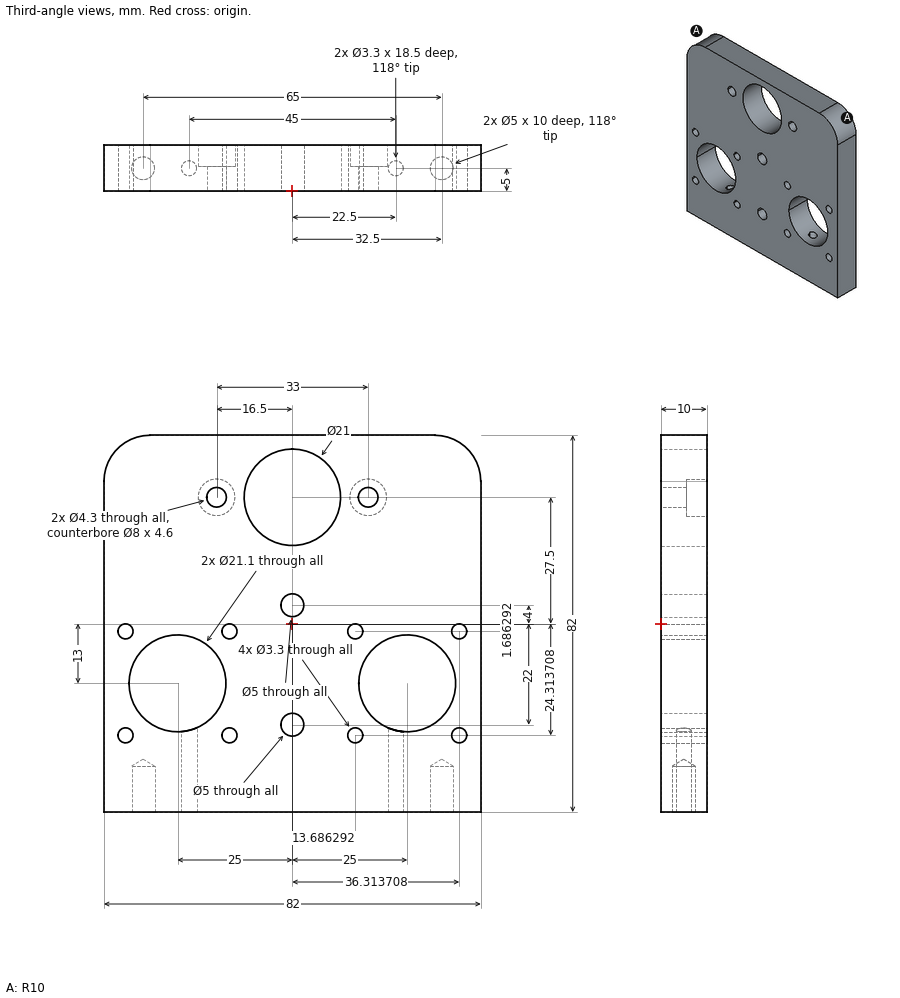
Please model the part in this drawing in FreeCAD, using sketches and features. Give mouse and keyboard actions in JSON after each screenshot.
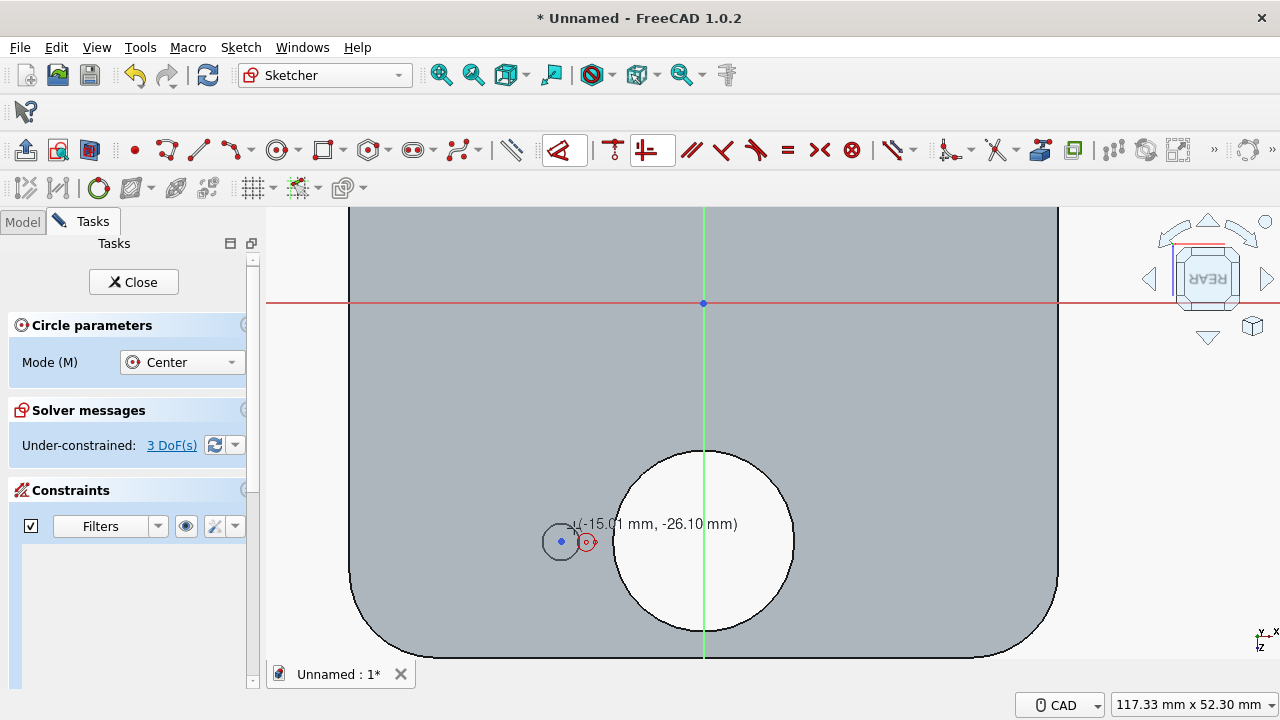
{"action": "left_click", "coordinate": [846, 541]}
{"action": "left_click", "coordinate": [859, 528]}
{"action": "key", "text": "Escape"}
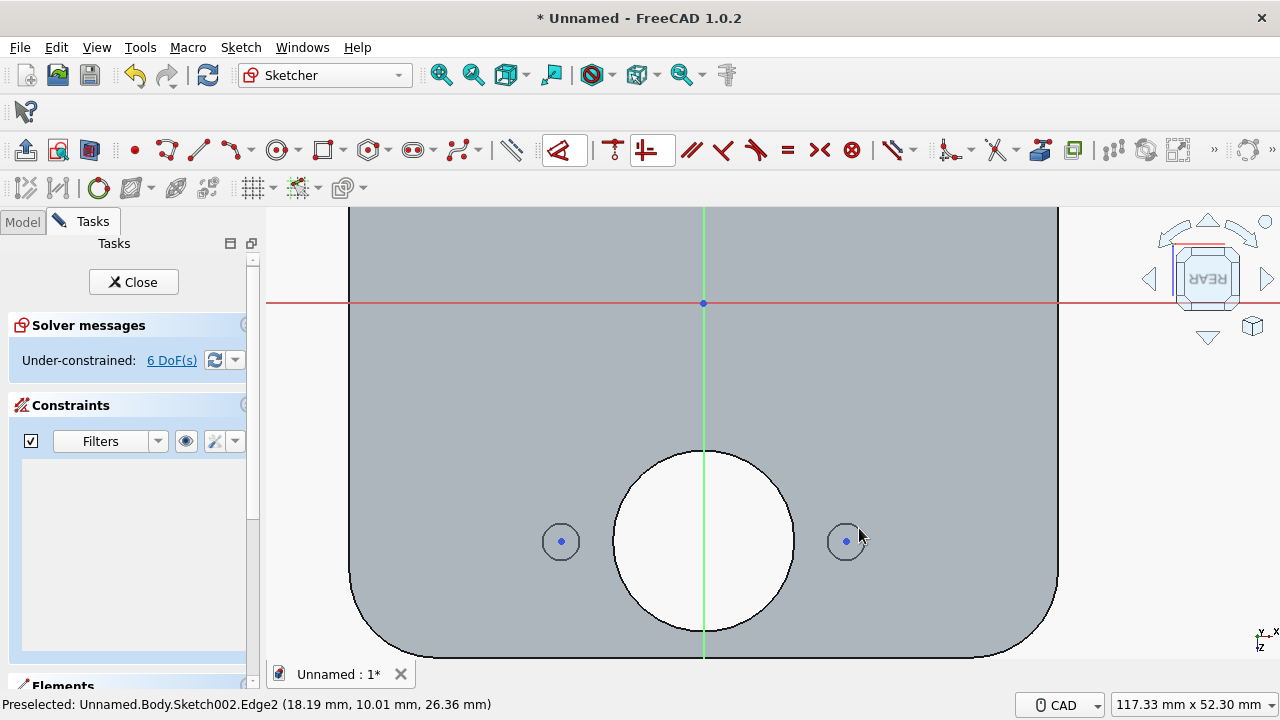
{"action": "left_click", "coordinate": [574, 529]}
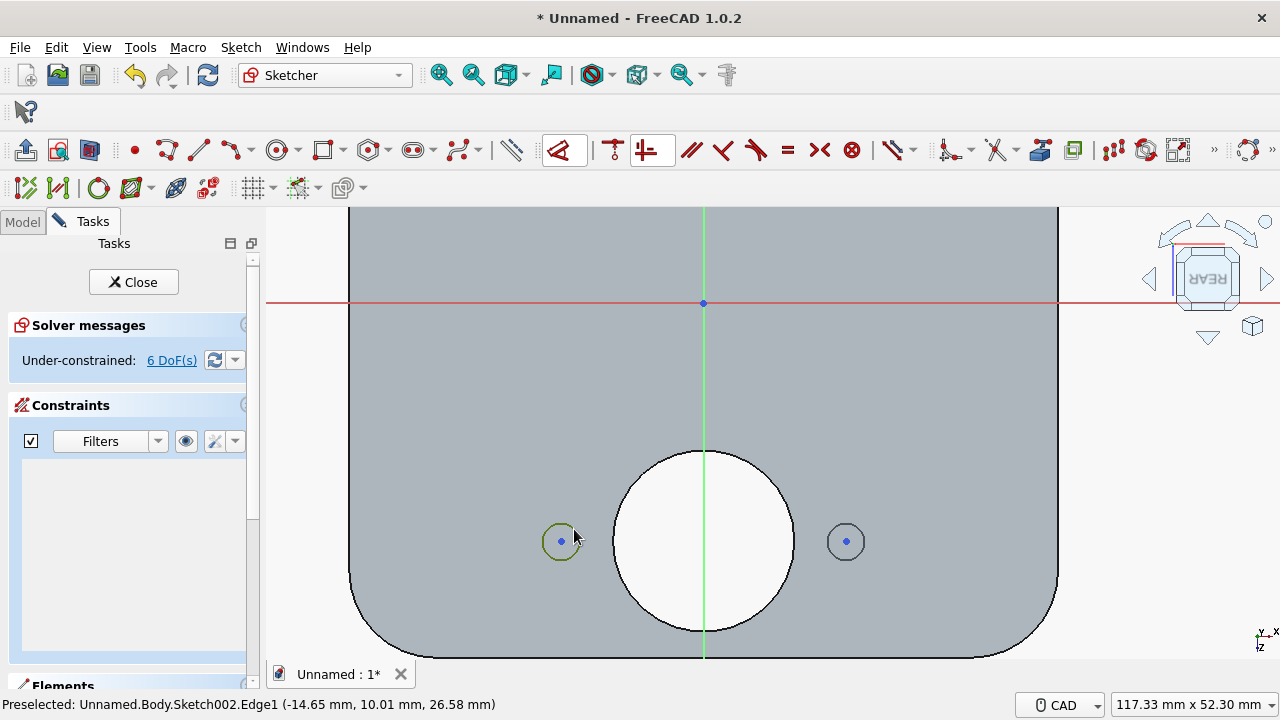
{"action": "left_click", "coordinate": [859, 529]}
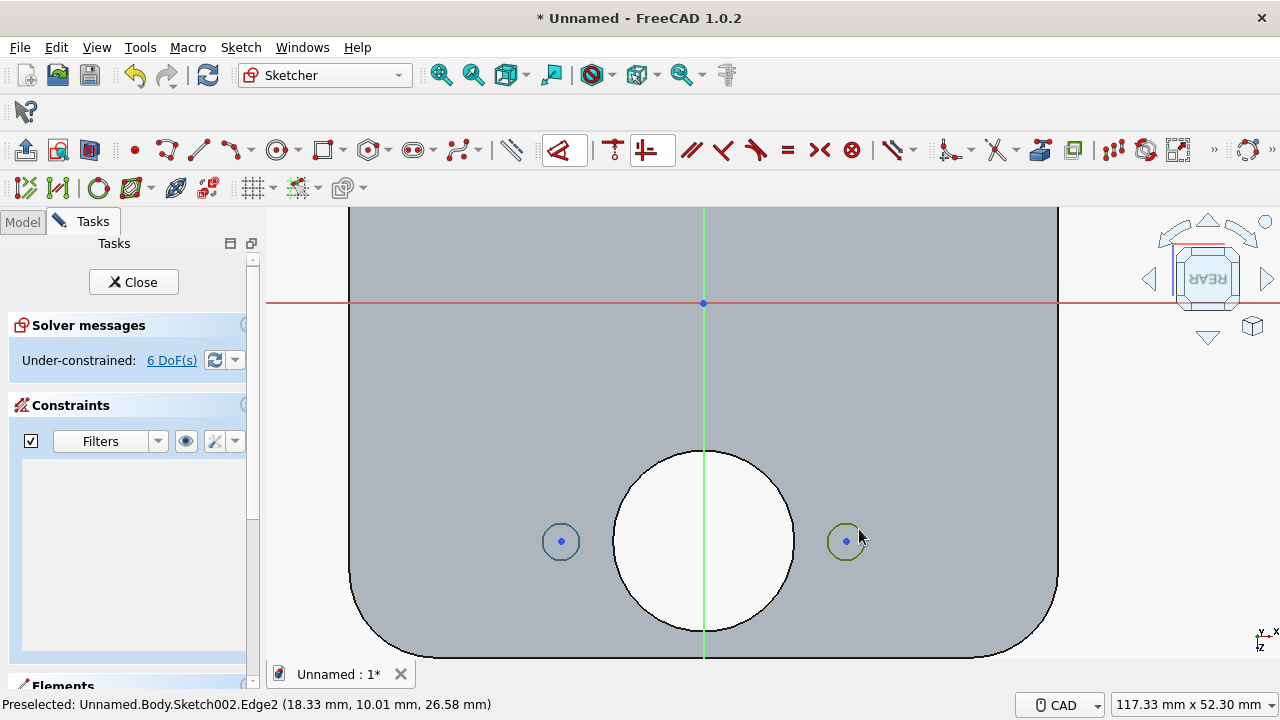
{"action": "left_click", "coordinate": [788, 150]}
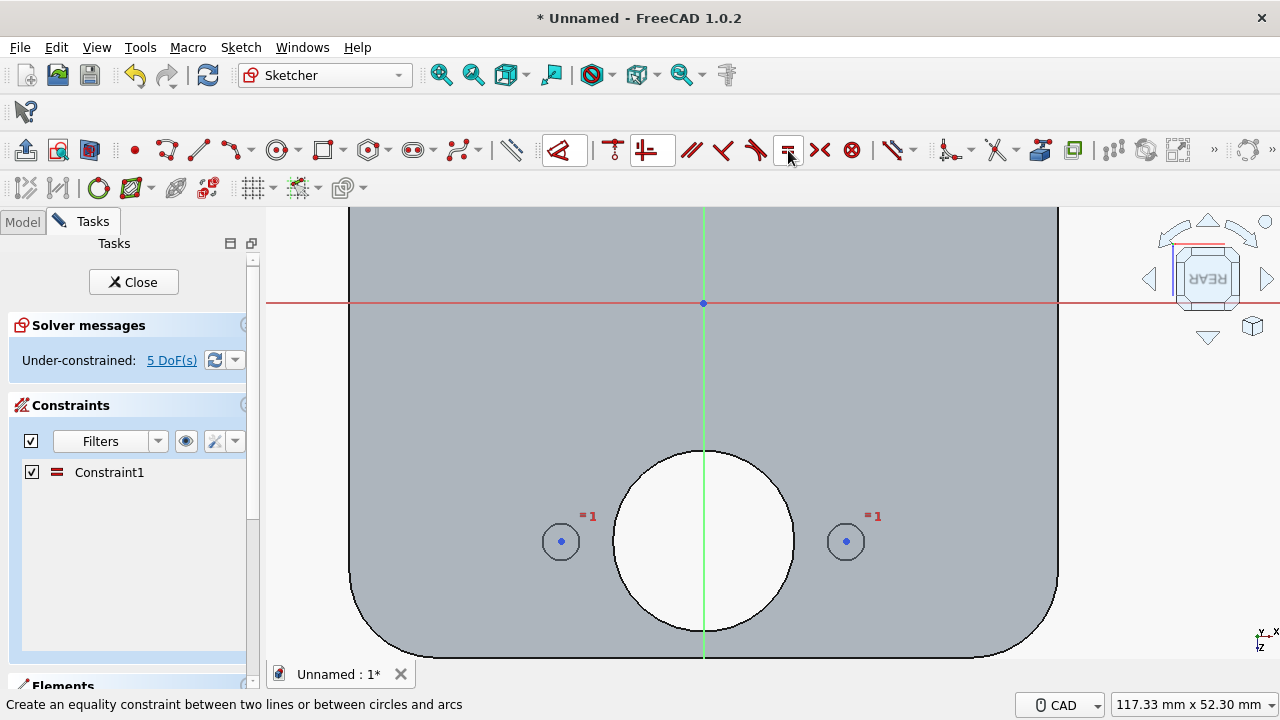
{"action": "left_click", "coordinate": [574, 529]}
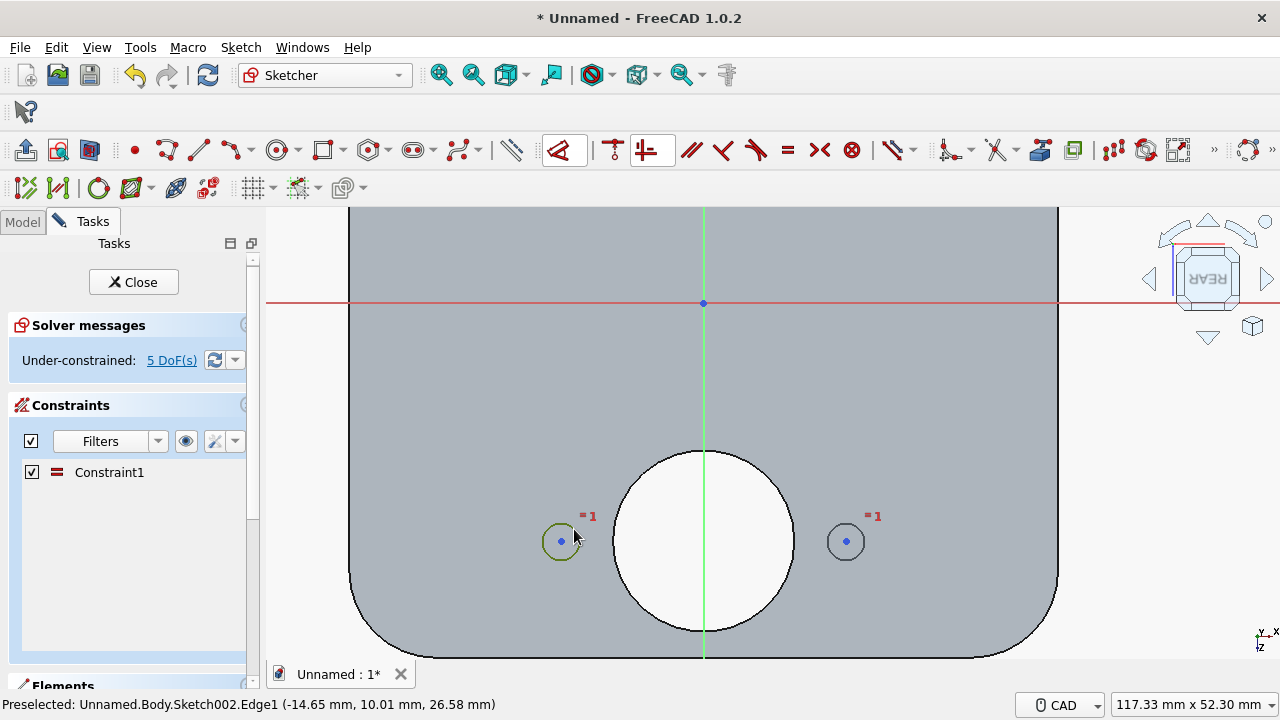
{"action": "left_click", "coordinate": [582, 150]}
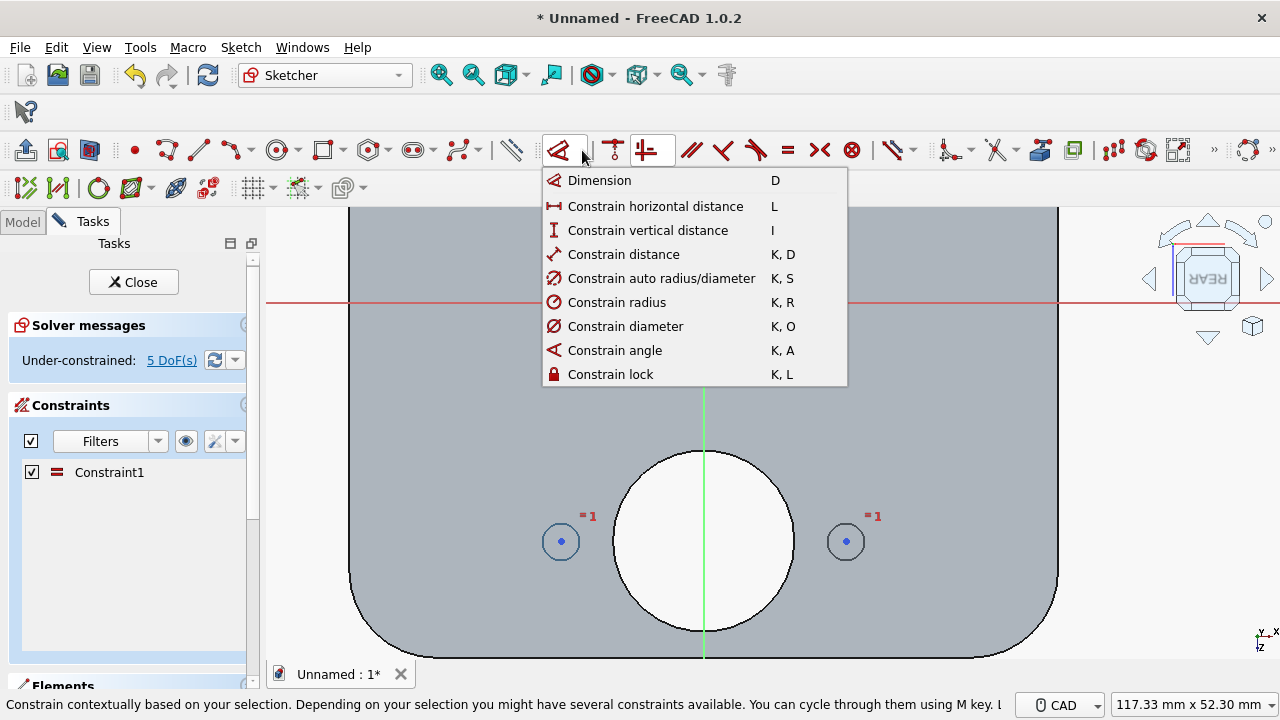
{"action": "left_click", "coordinate": [695, 326]}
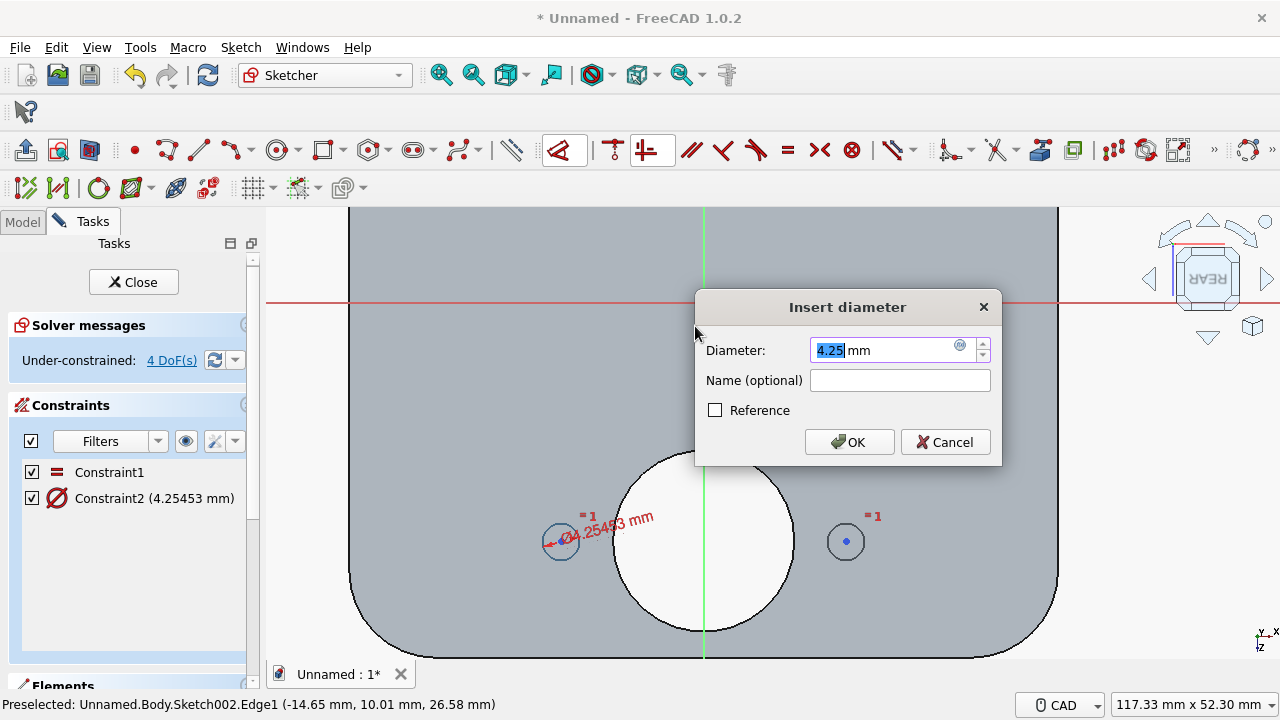
{"action": "type", "text": "4.3"}
{"action": "key", "text": "Return"}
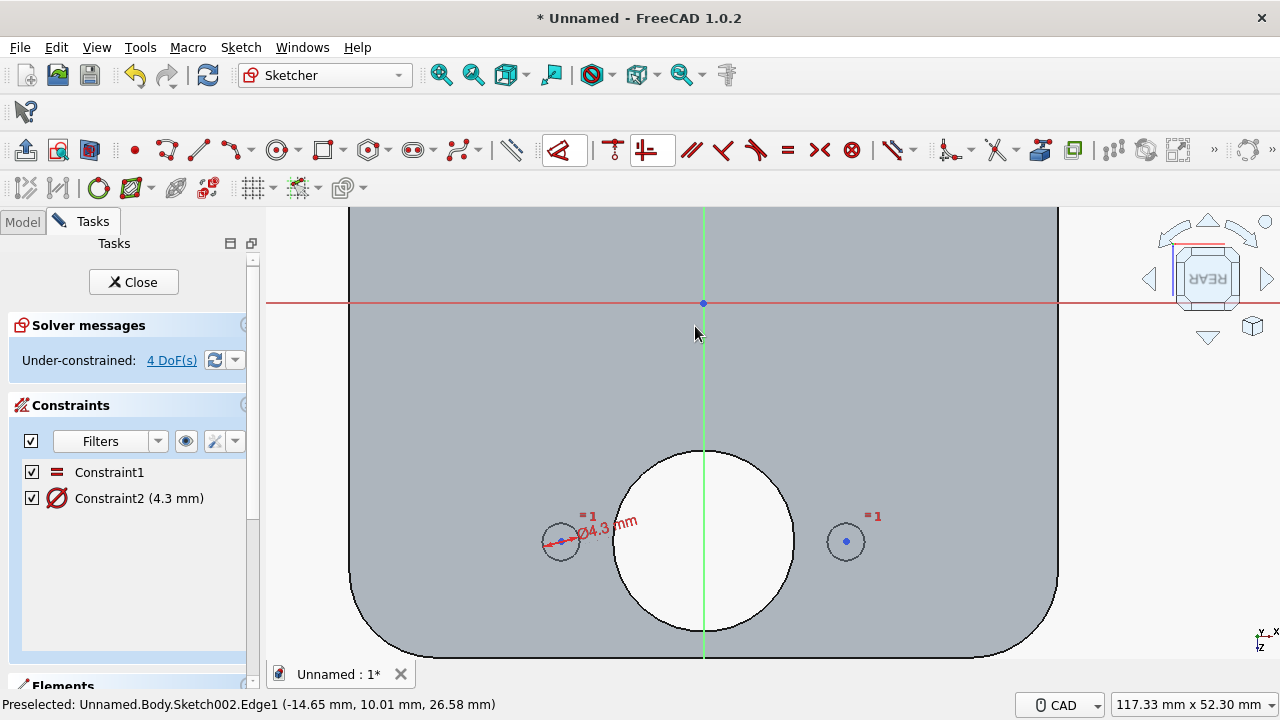
{"action": "left_click", "coordinate": [561, 542]}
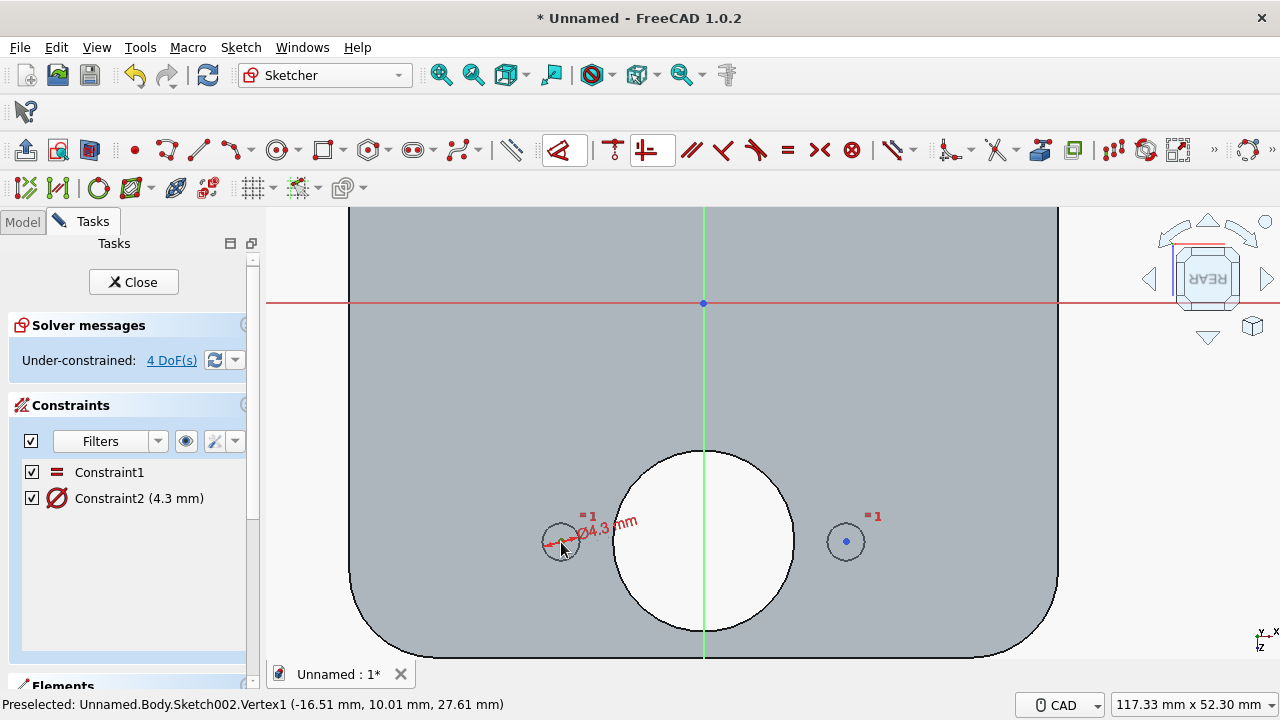
{"action": "left_click", "coordinate": [846, 542]}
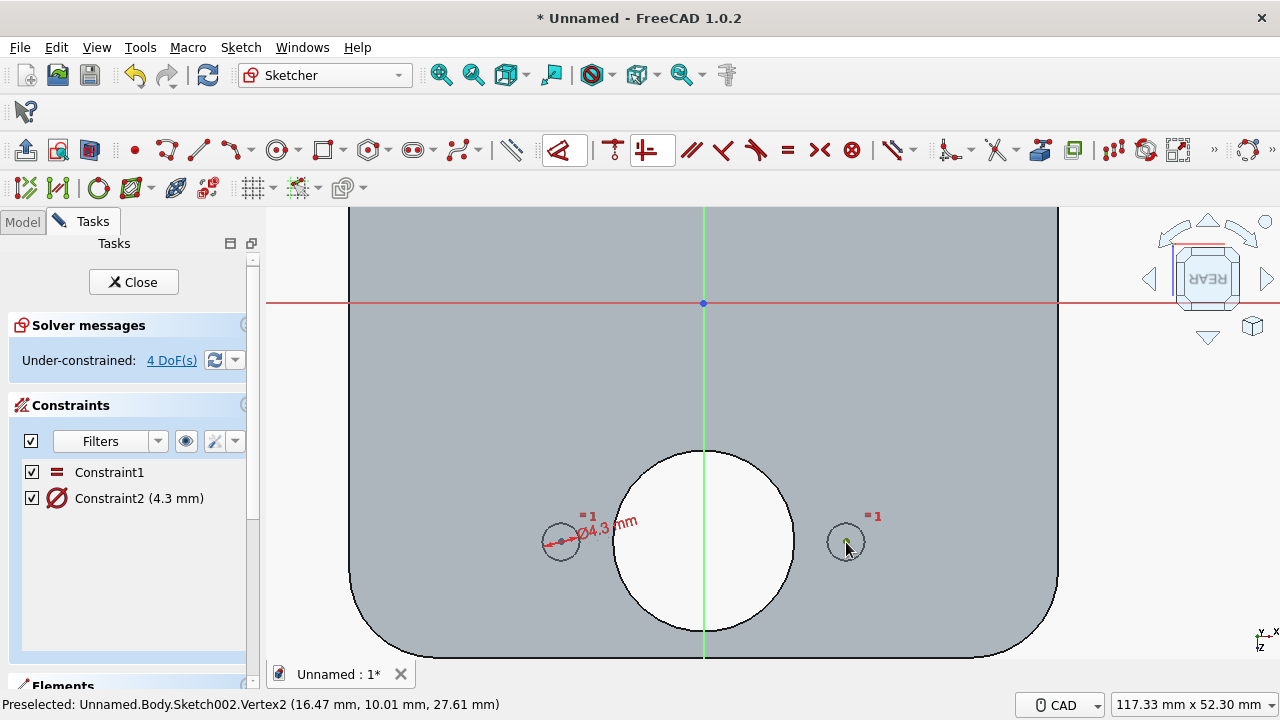
{"action": "left_click", "coordinate": [582, 150]}